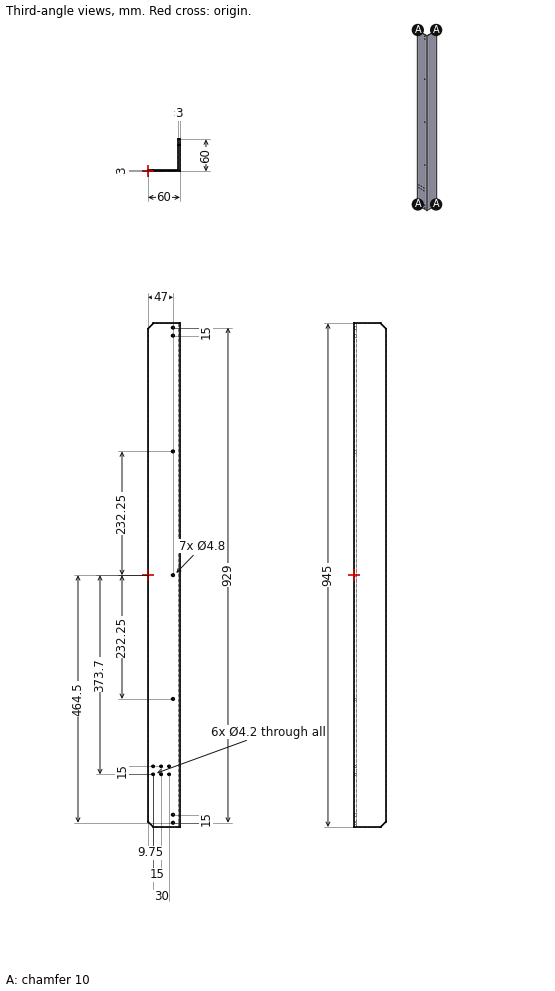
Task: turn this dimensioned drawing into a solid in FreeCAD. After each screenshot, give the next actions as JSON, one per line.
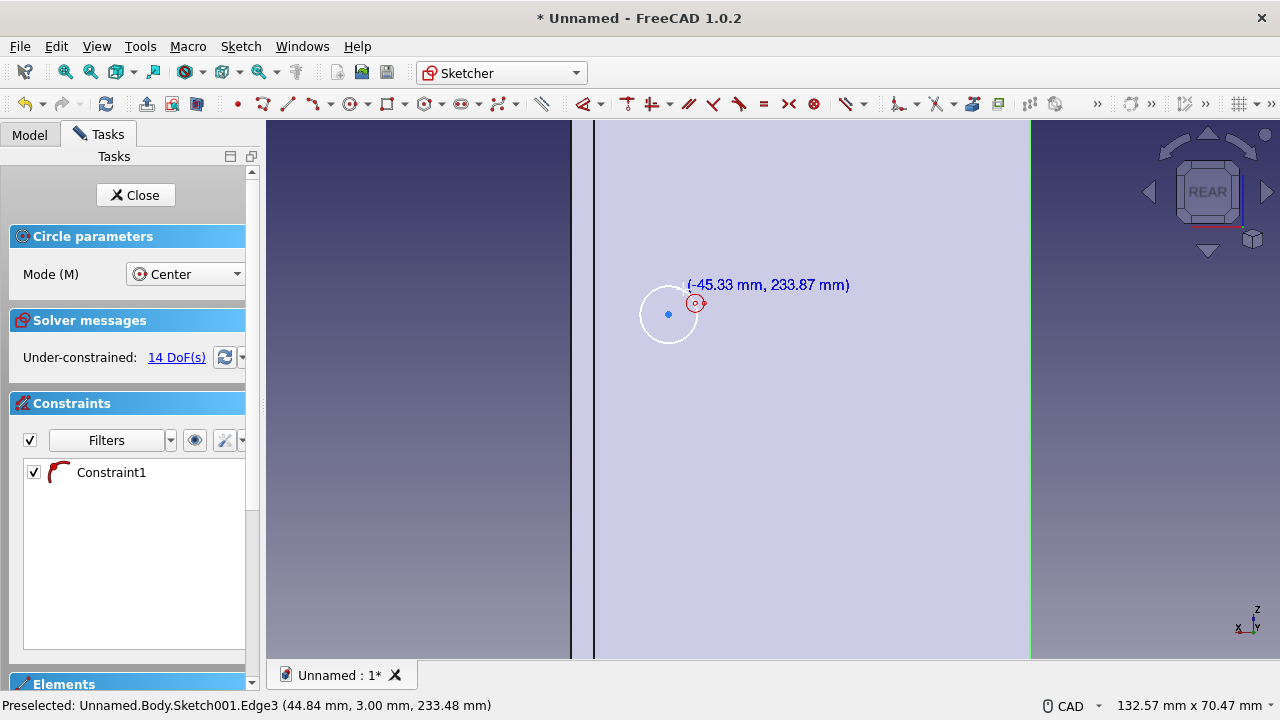
{"action": "scroll", "coordinate": [697, 301], "scroll_direction": "down", "scroll_amount": 15}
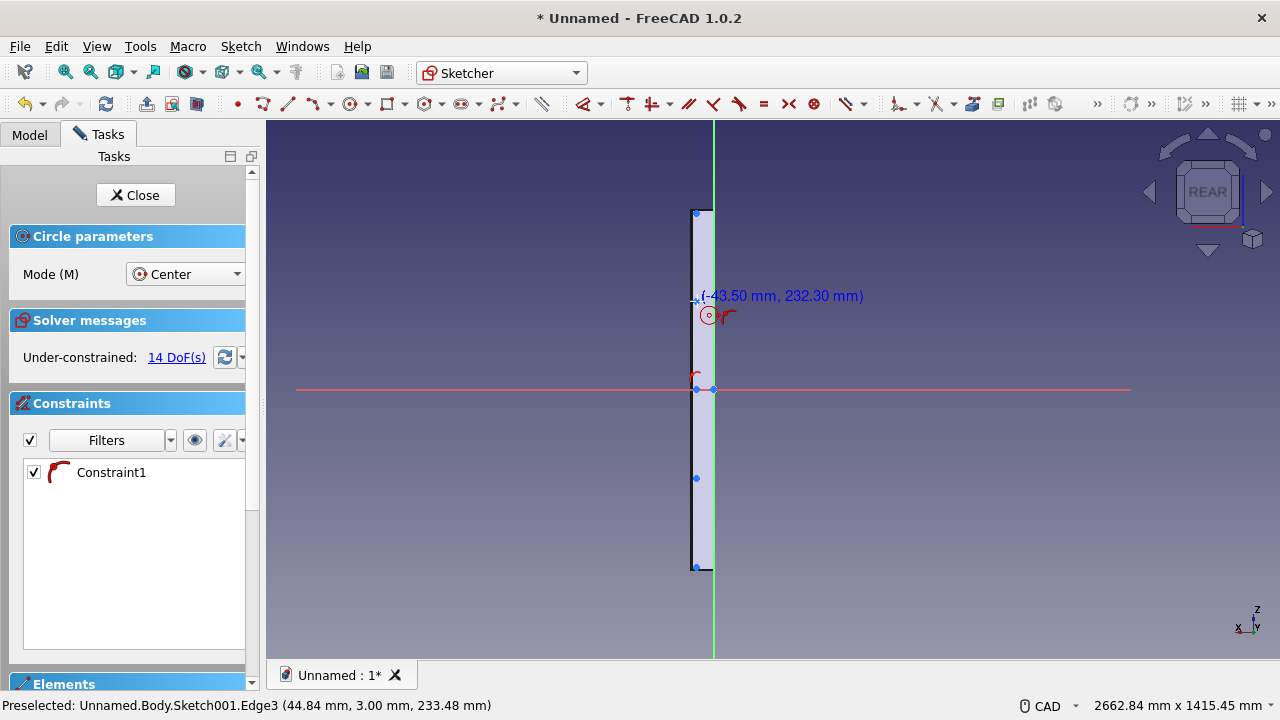
{"action": "scroll", "coordinate": [696, 561], "scroll_direction": "up", "scroll_amount": 17}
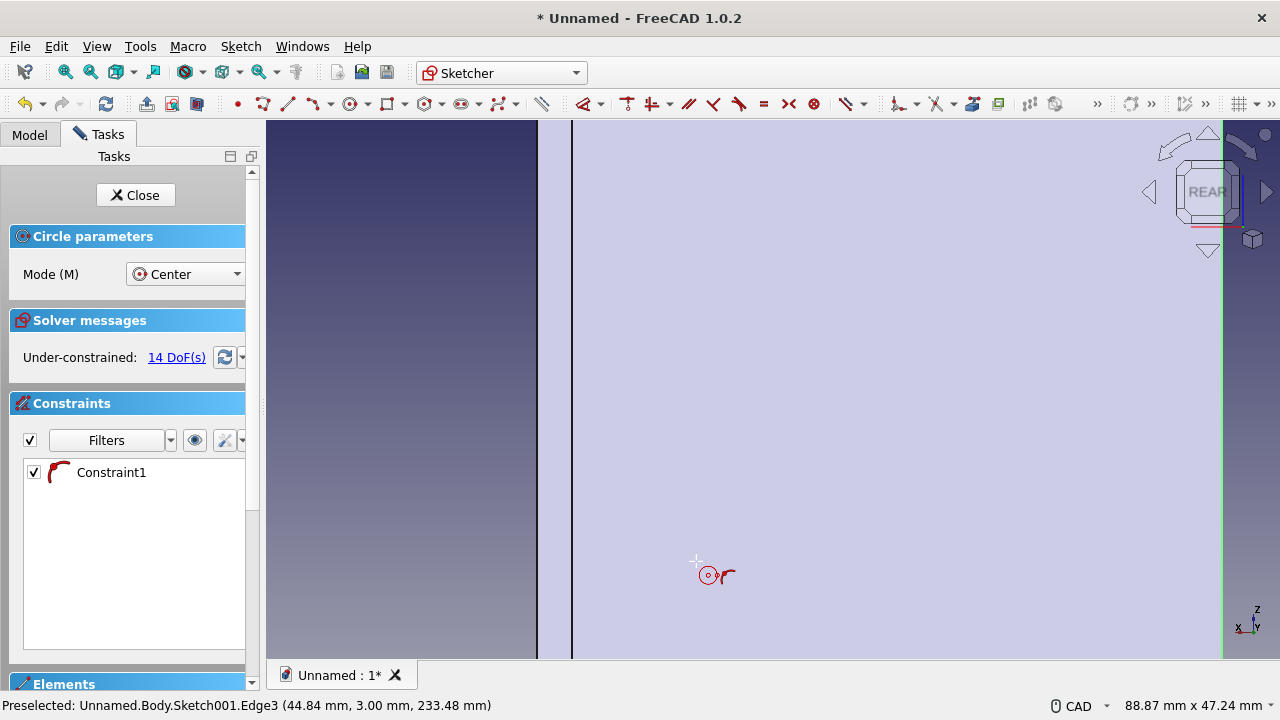
{"action": "scroll", "coordinate": [696, 561], "scroll_direction": "down", "scroll_amount": 17}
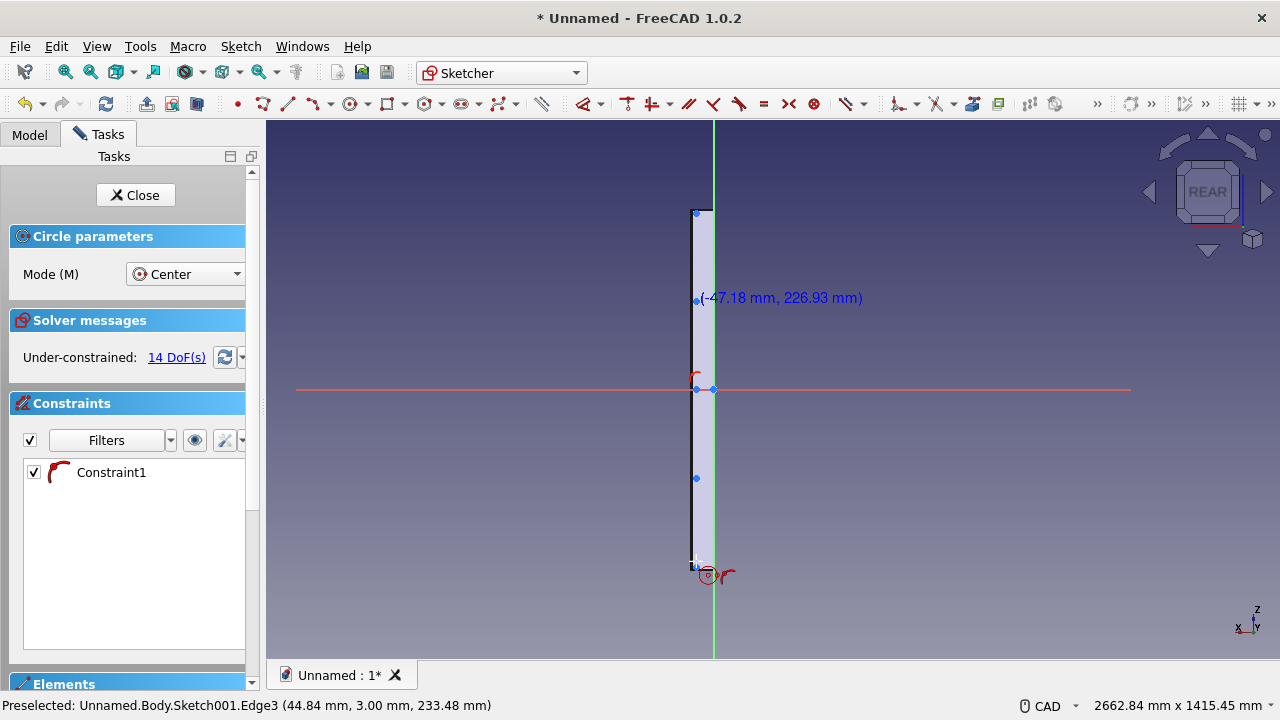
{"action": "scroll", "coordinate": [696, 561], "scroll_direction": "up", "scroll_amount": 6}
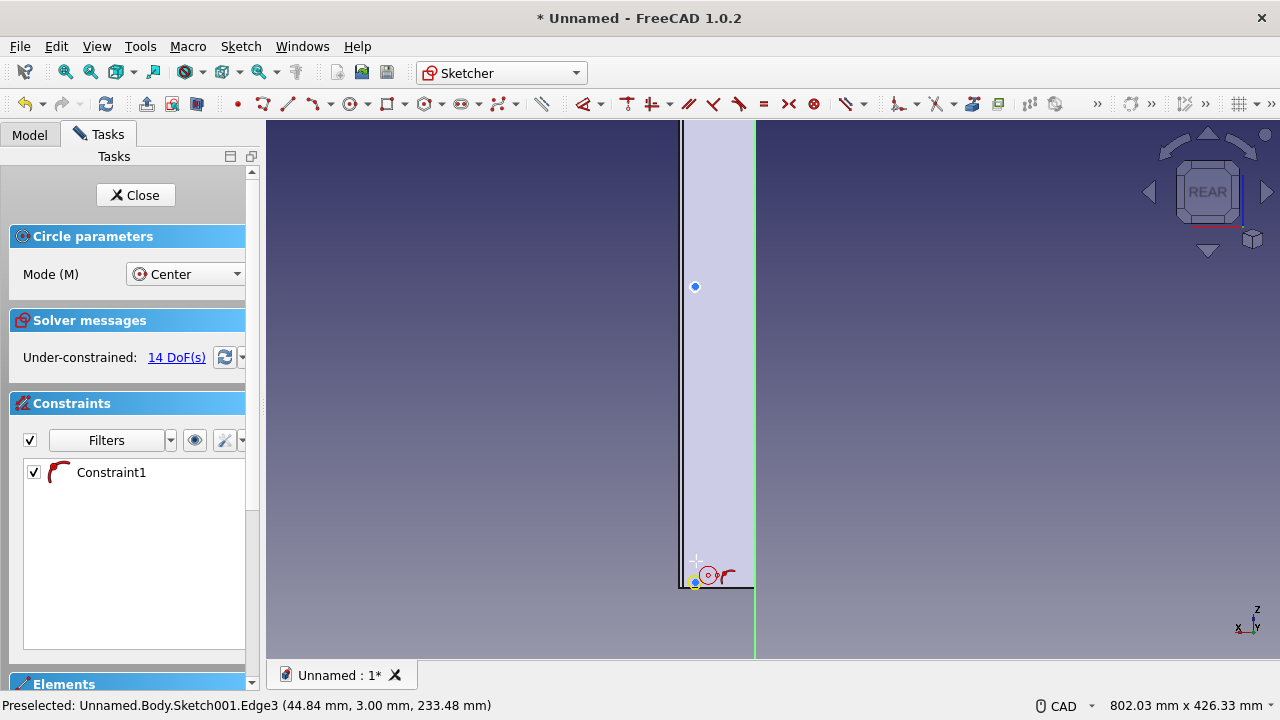
{"action": "left_click", "coordinate": [695, 559]}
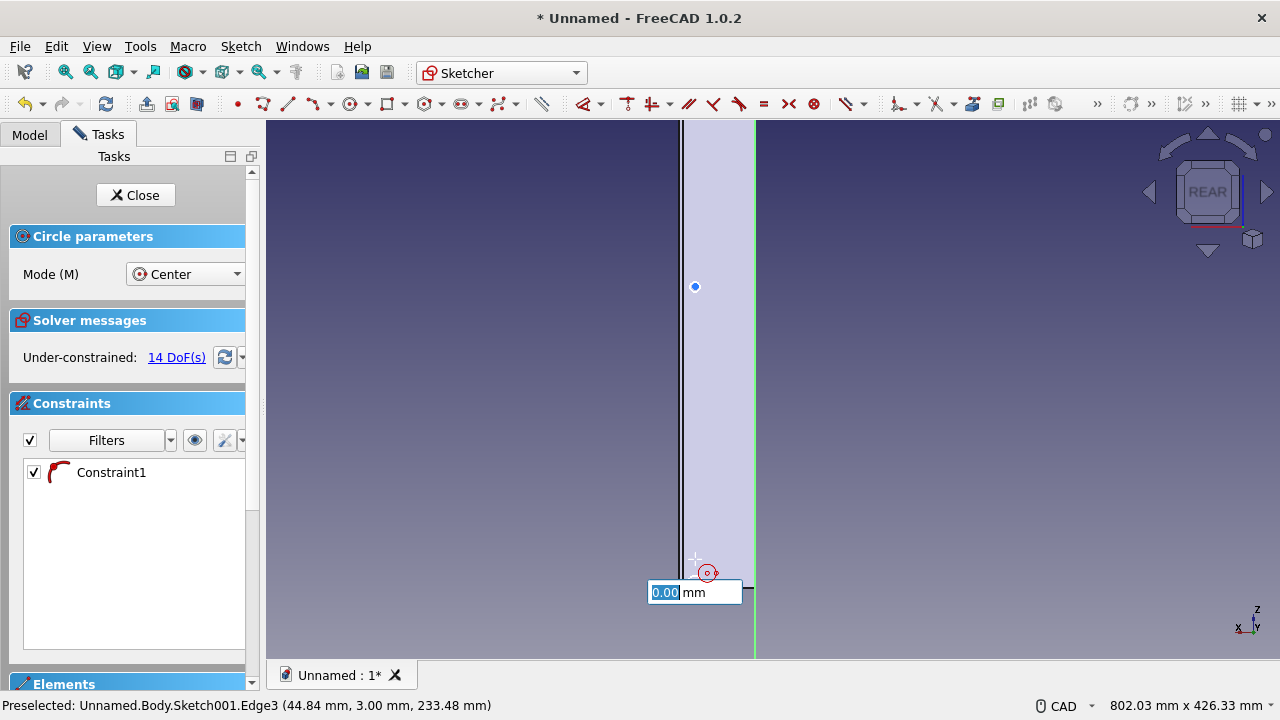
{"action": "scroll", "coordinate": [697, 557], "scroll_direction": "up", "scroll_amount": 9}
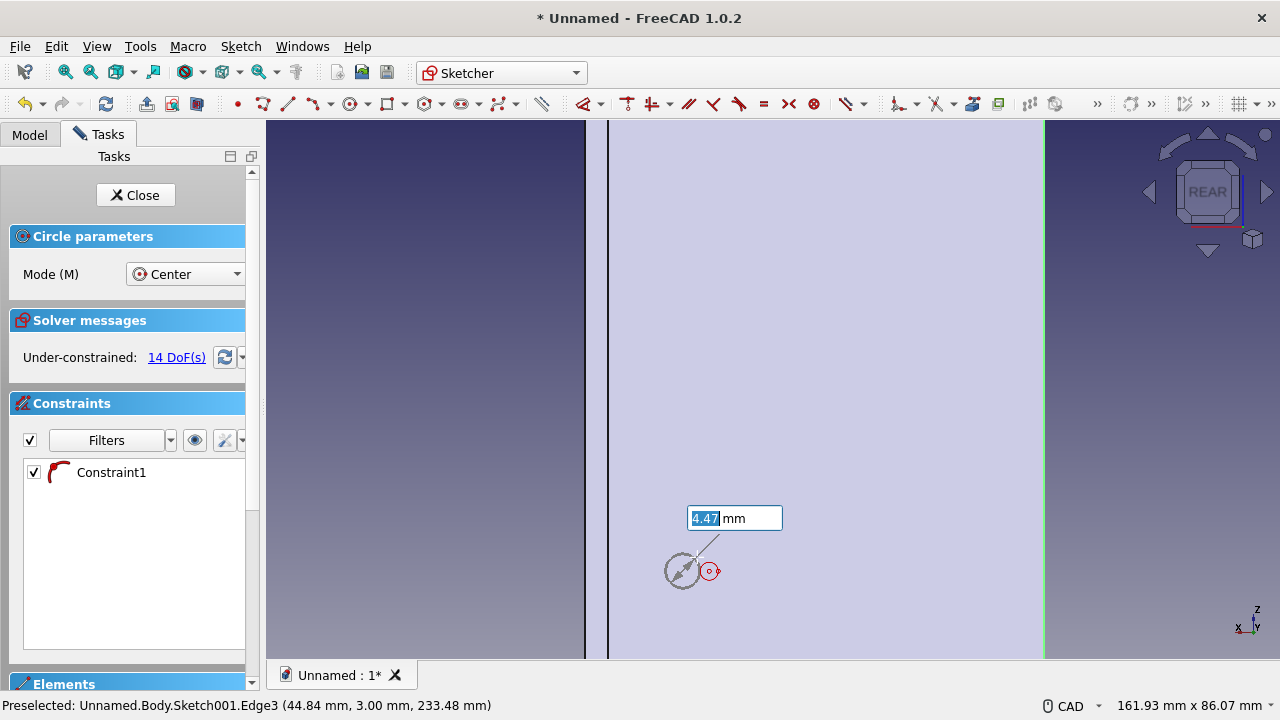
{"action": "left_click", "coordinate": [697, 553]}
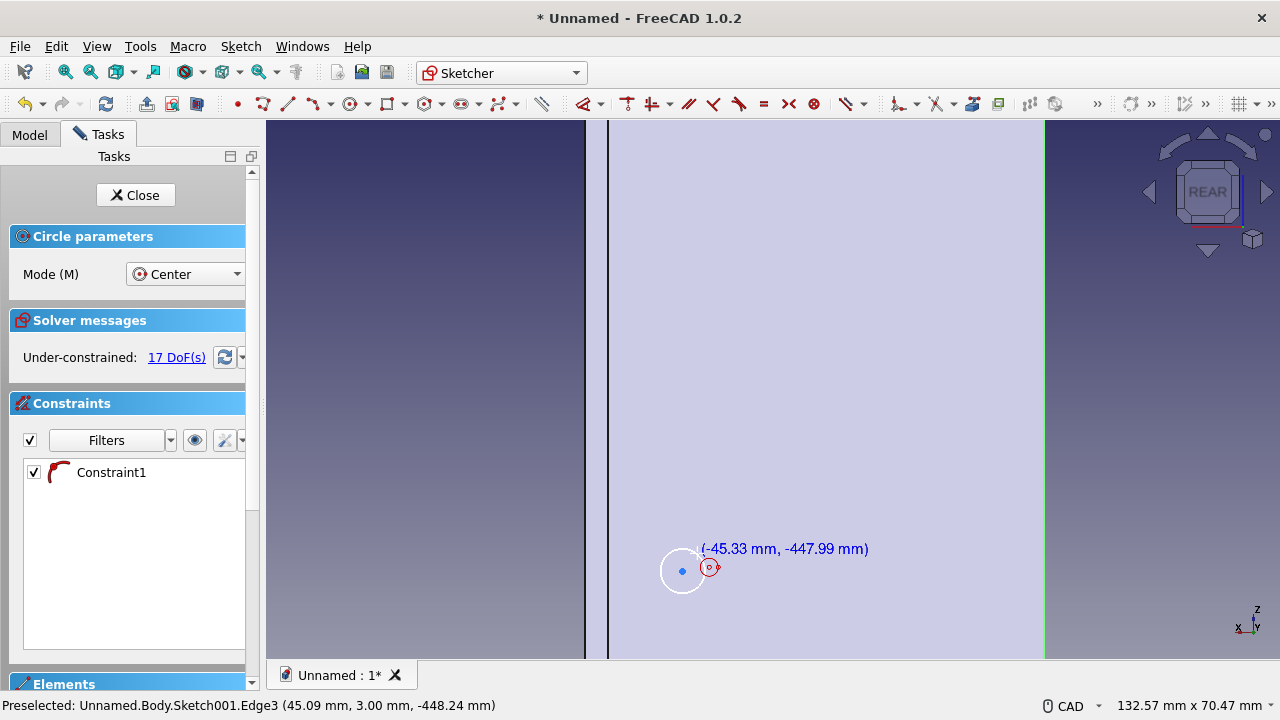
{"action": "scroll", "coordinate": [697, 560], "scroll_direction": "down", "scroll_amount": 15}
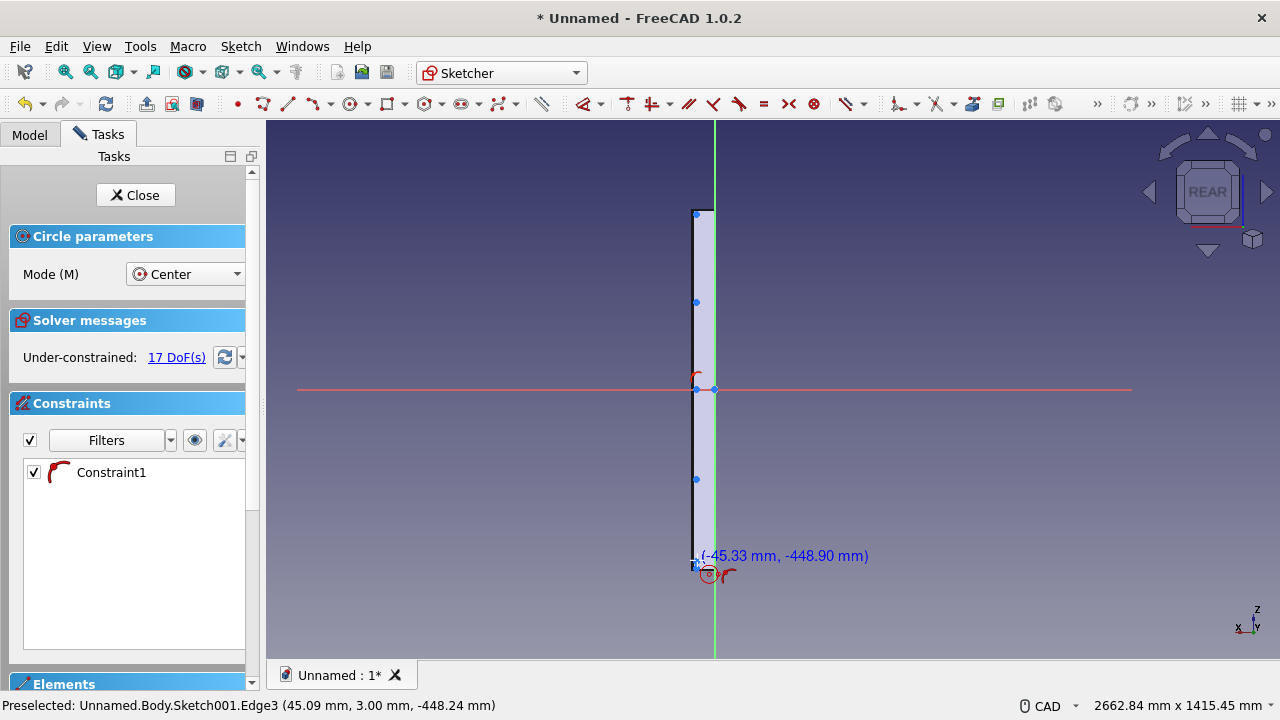
{"action": "scroll", "coordinate": [697, 219], "scroll_direction": "up", "scroll_amount": 17}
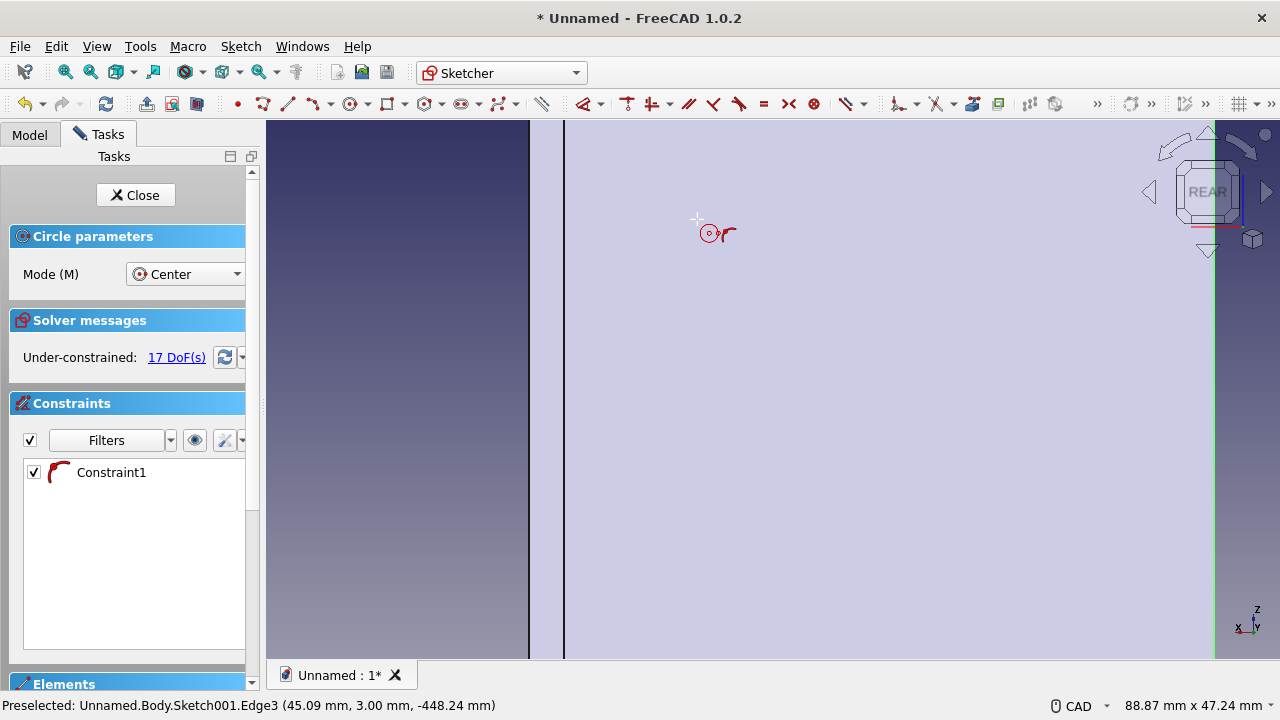
{"action": "scroll", "coordinate": [697, 219], "scroll_direction": "down", "scroll_amount": 17}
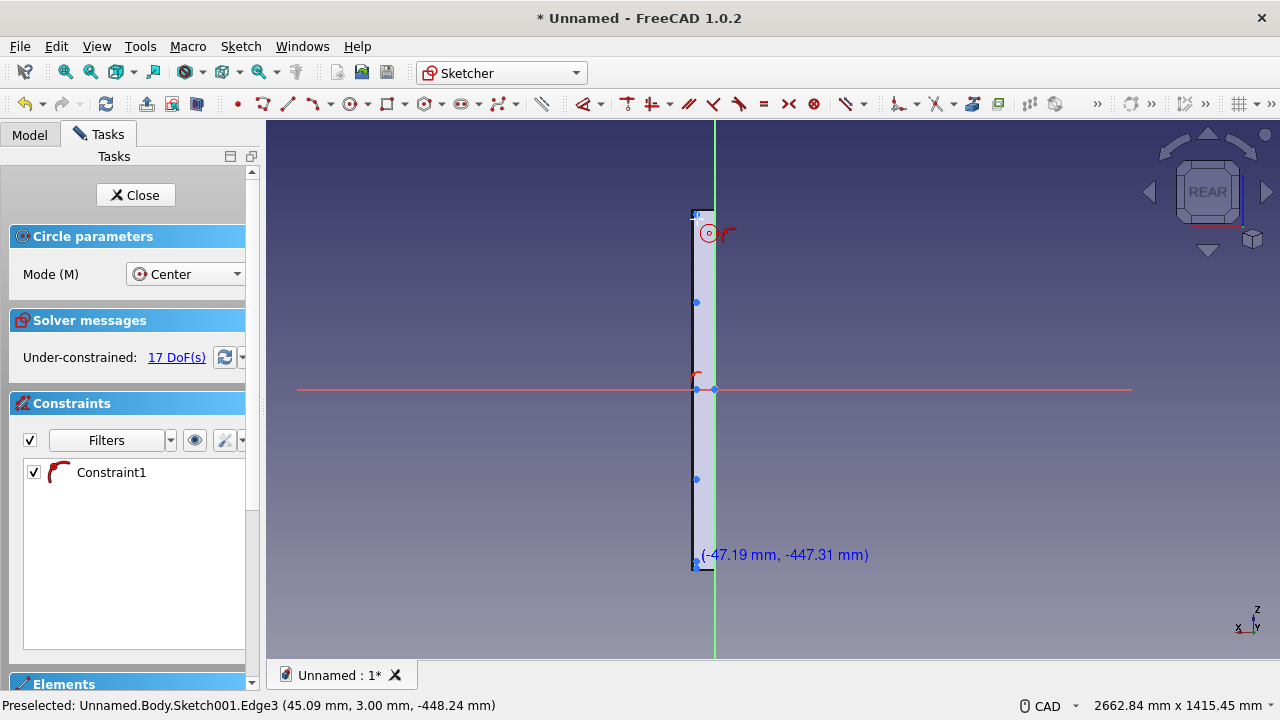
{"action": "scroll", "coordinate": [697, 219], "scroll_direction": "up", "scroll_amount": 6}